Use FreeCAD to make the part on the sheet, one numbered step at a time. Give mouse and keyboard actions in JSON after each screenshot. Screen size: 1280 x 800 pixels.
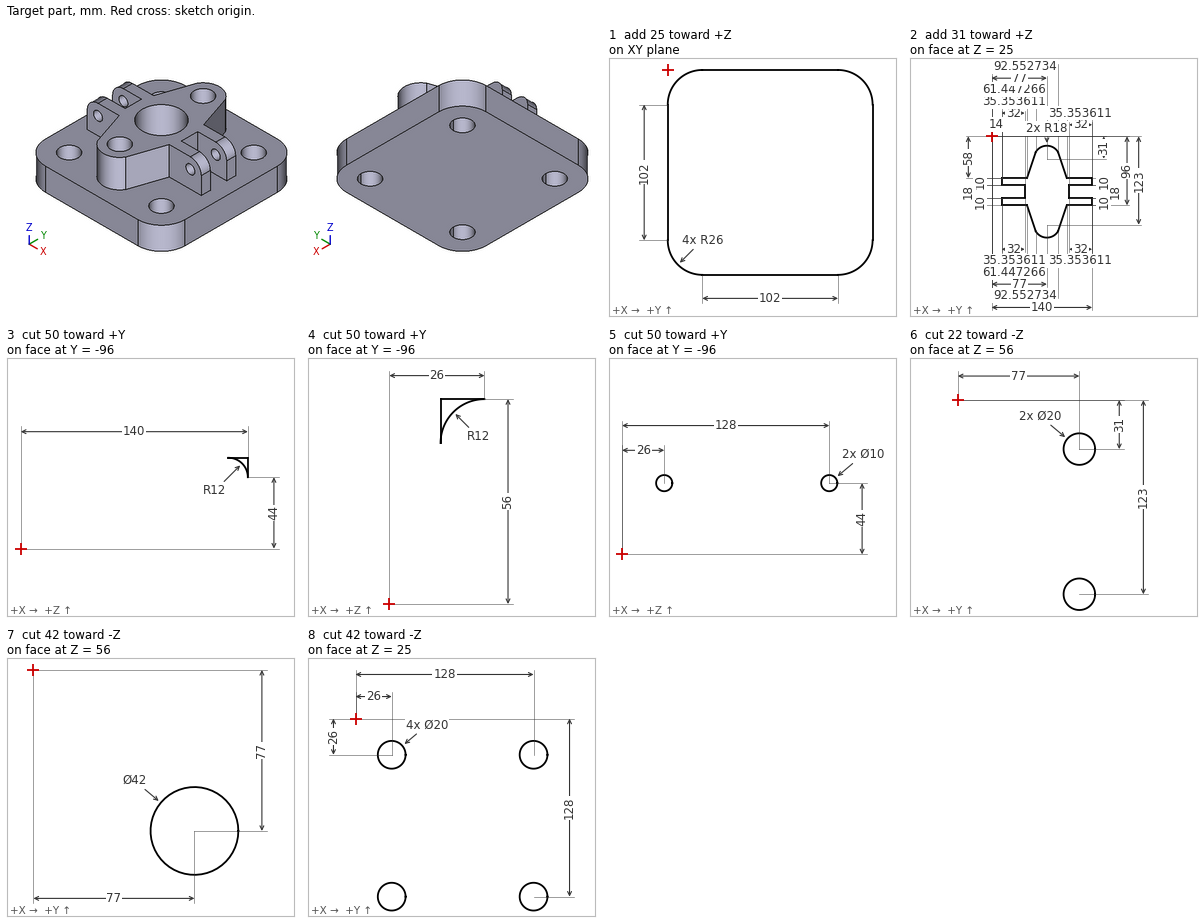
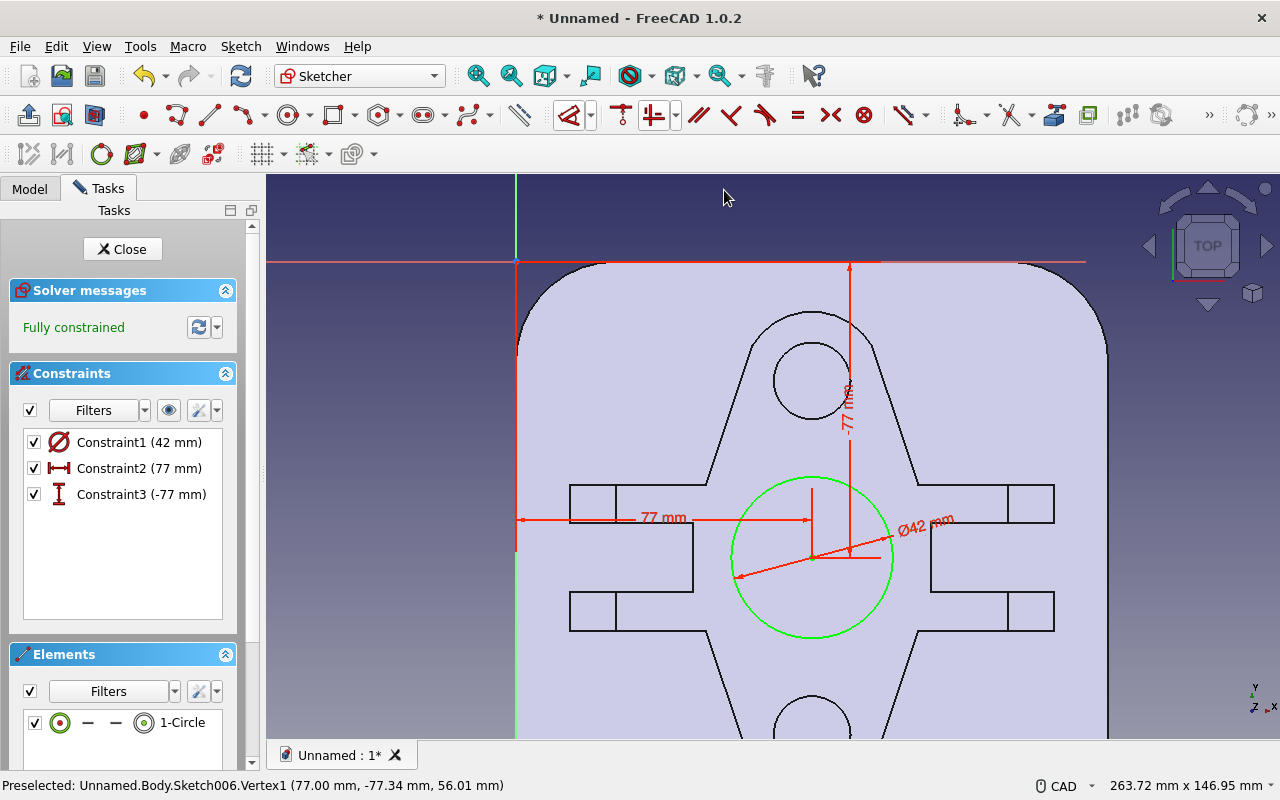
{"action": "left_click", "coordinate": [123, 249]}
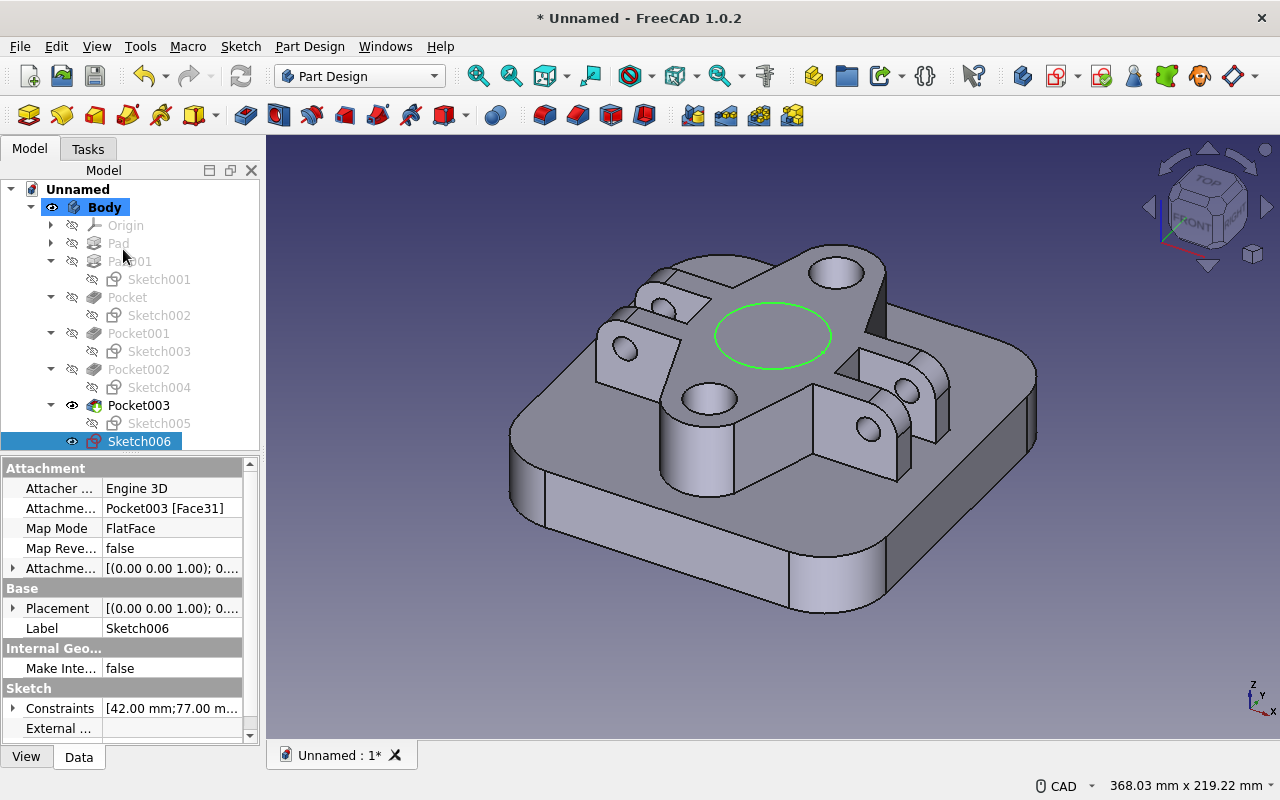
{"action": "left_click", "coordinate": [246, 116]}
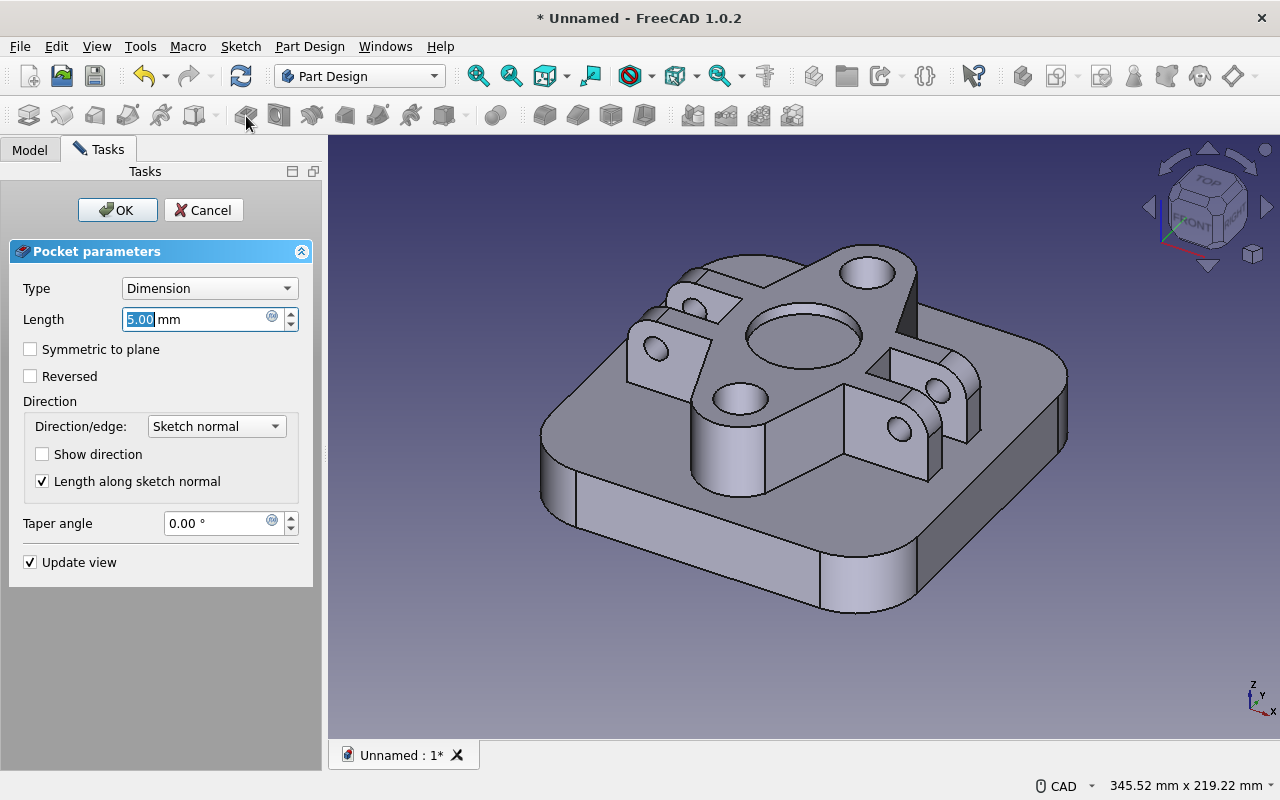
{"action": "type", "text": "42"}
{"action": "key", "text": "Tab"}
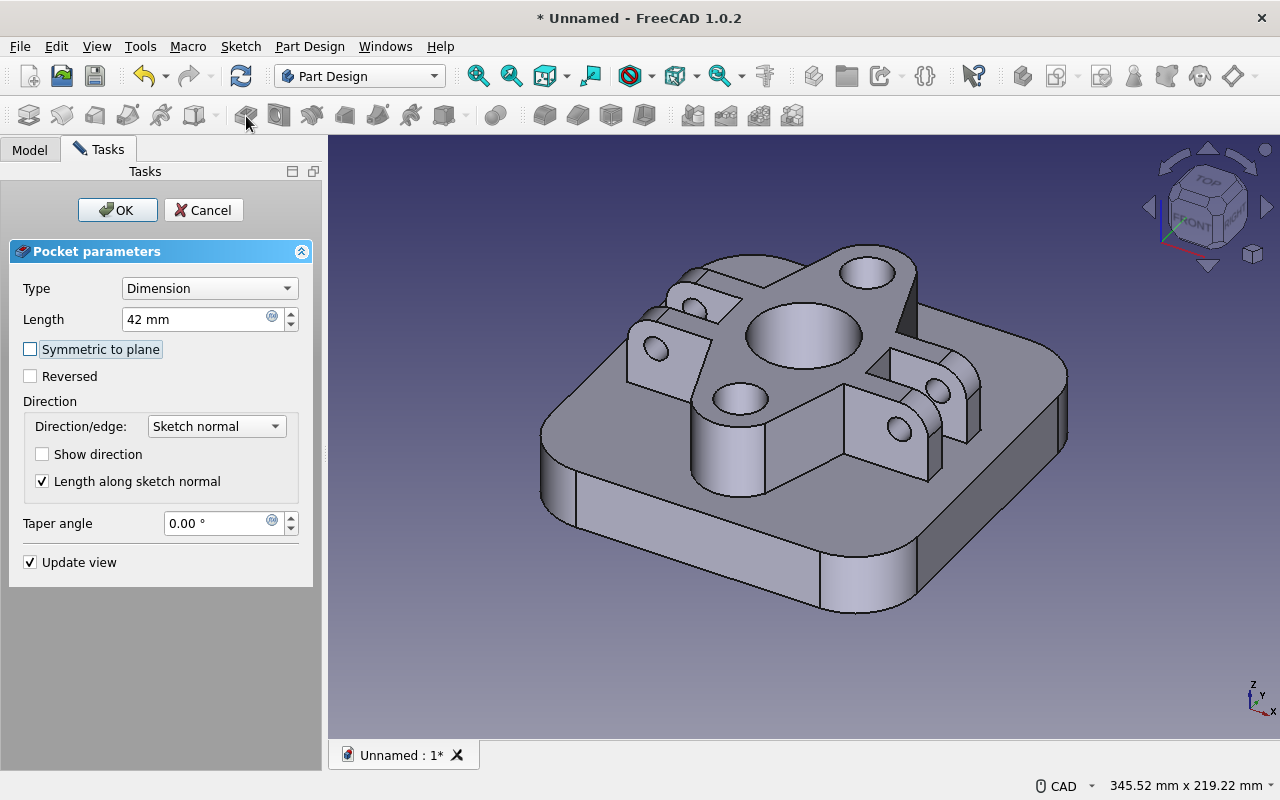
{"action": "left_click", "coordinate": [118, 210]}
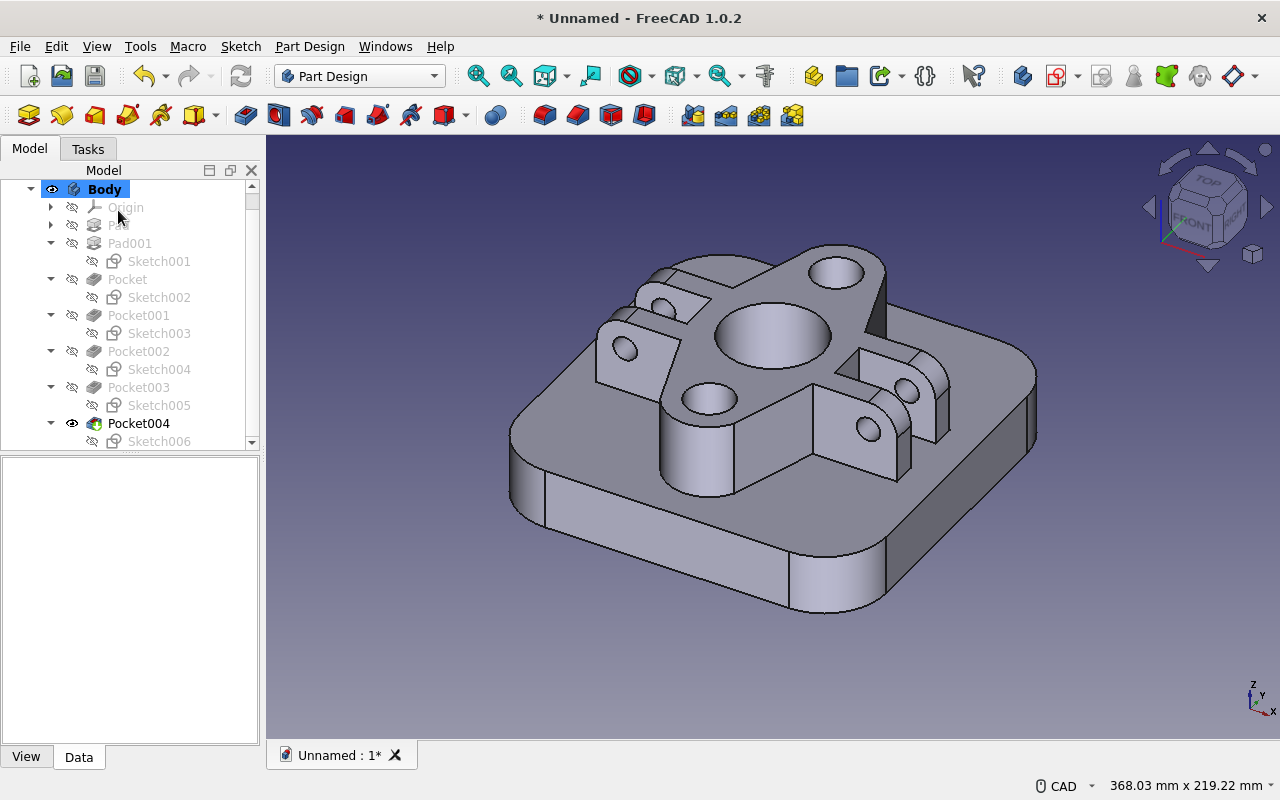
{"action": "left_click", "coordinate": [607, 430]}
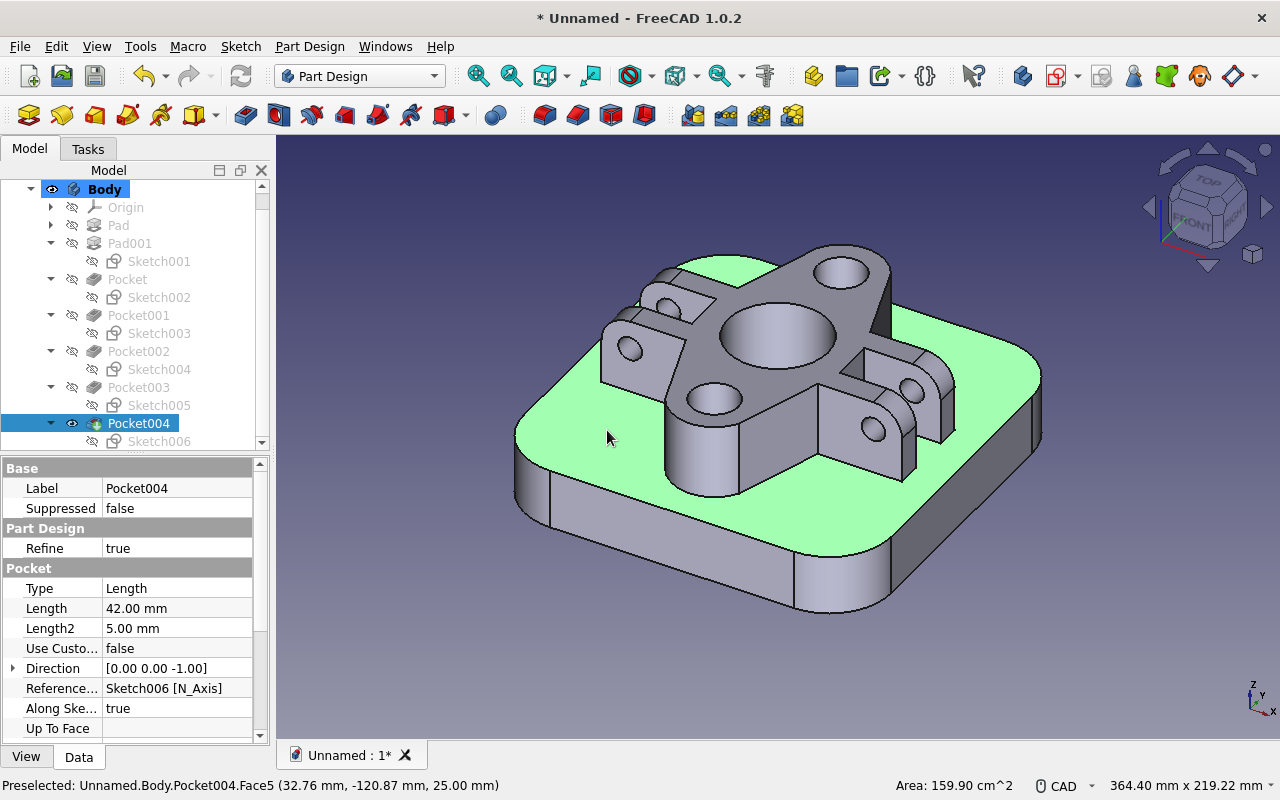
{"action": "left_click", "coordinate": [1056, 76]}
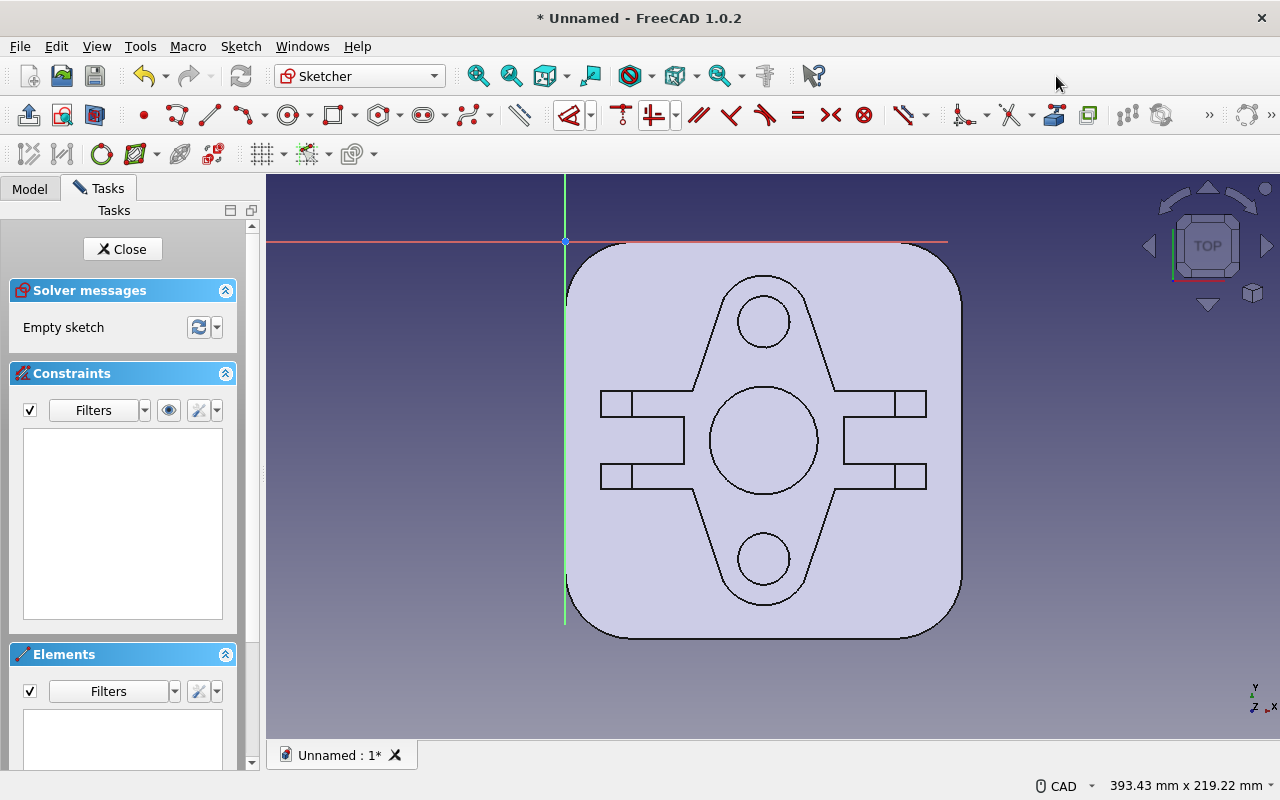
{"action": "left_click", "coordinate": [288, 116]}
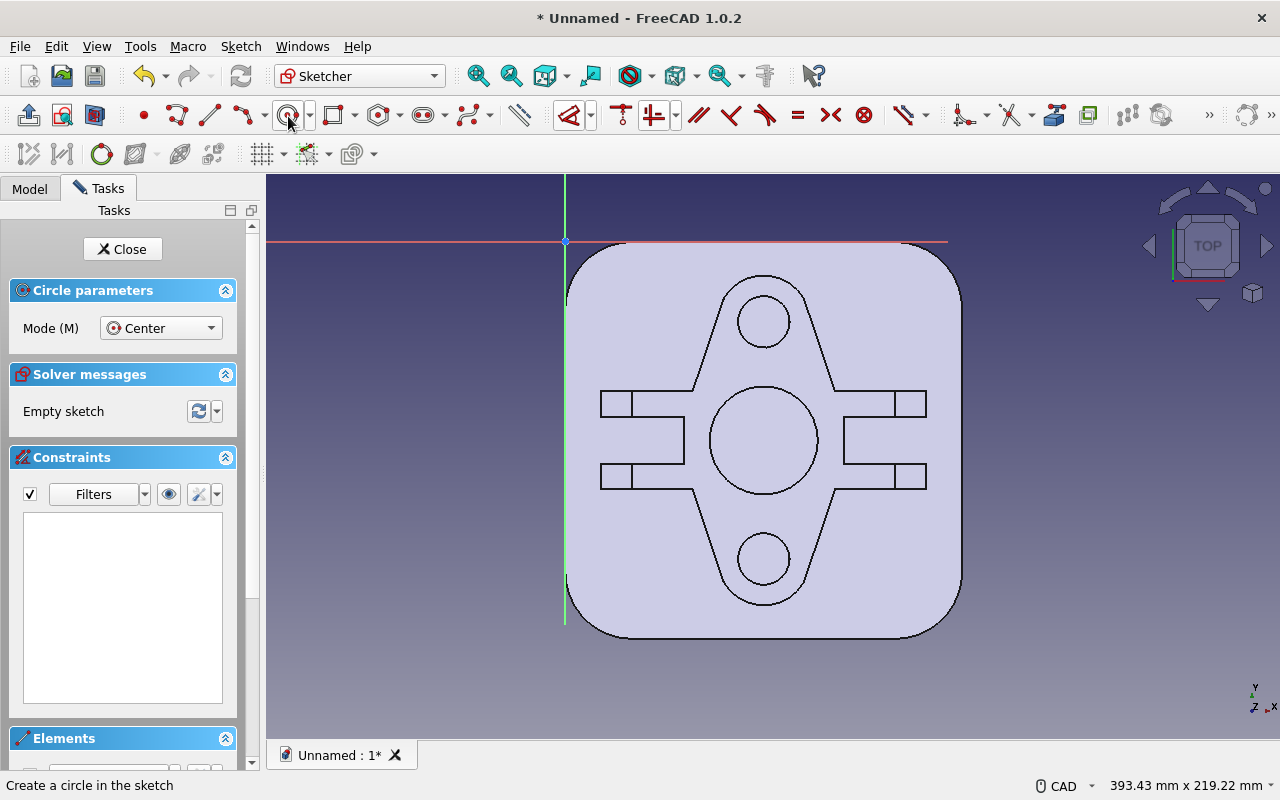
{"action": "left_click", "coordinate": [632, 309]}
{"action": "left_click", "coordinate": [651, 291]}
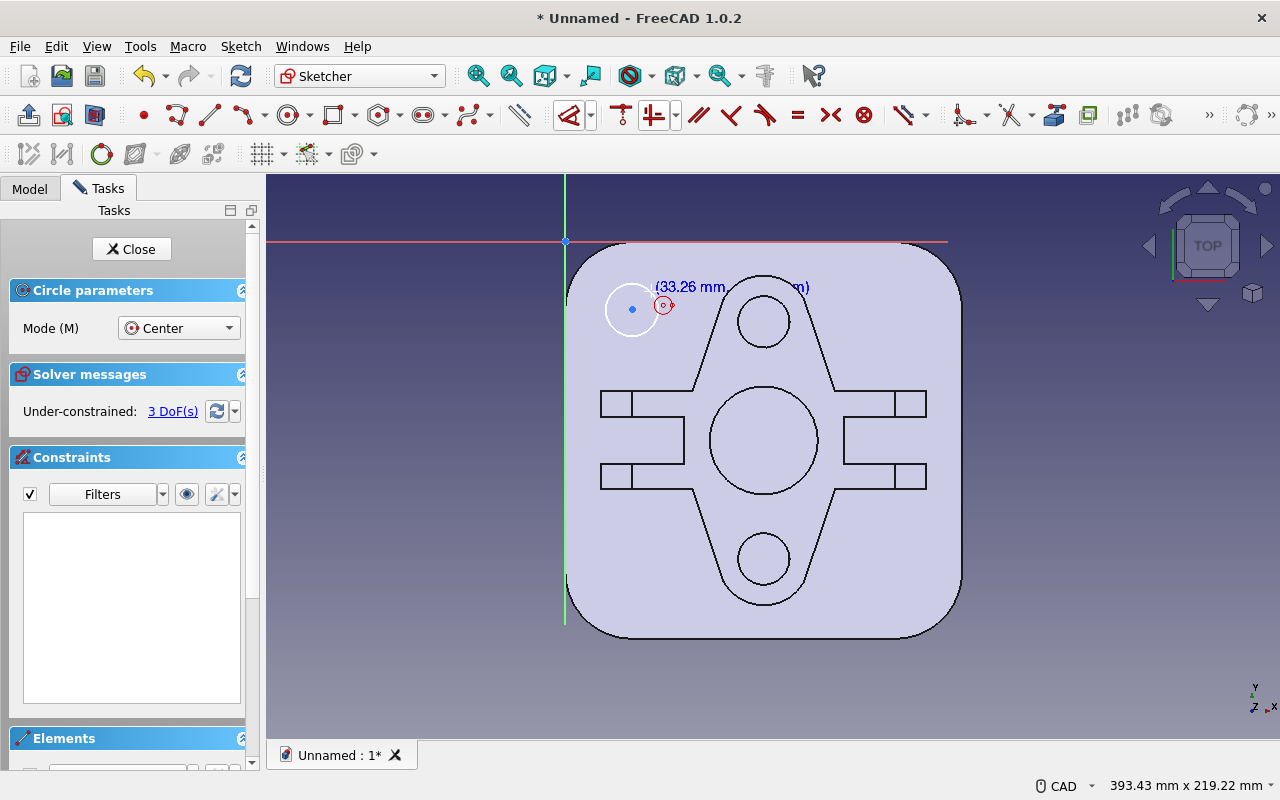
{"action": "left_click", "coordinate": [895, 309]}
{"action": "left_click", "coordinate": [913, 291]}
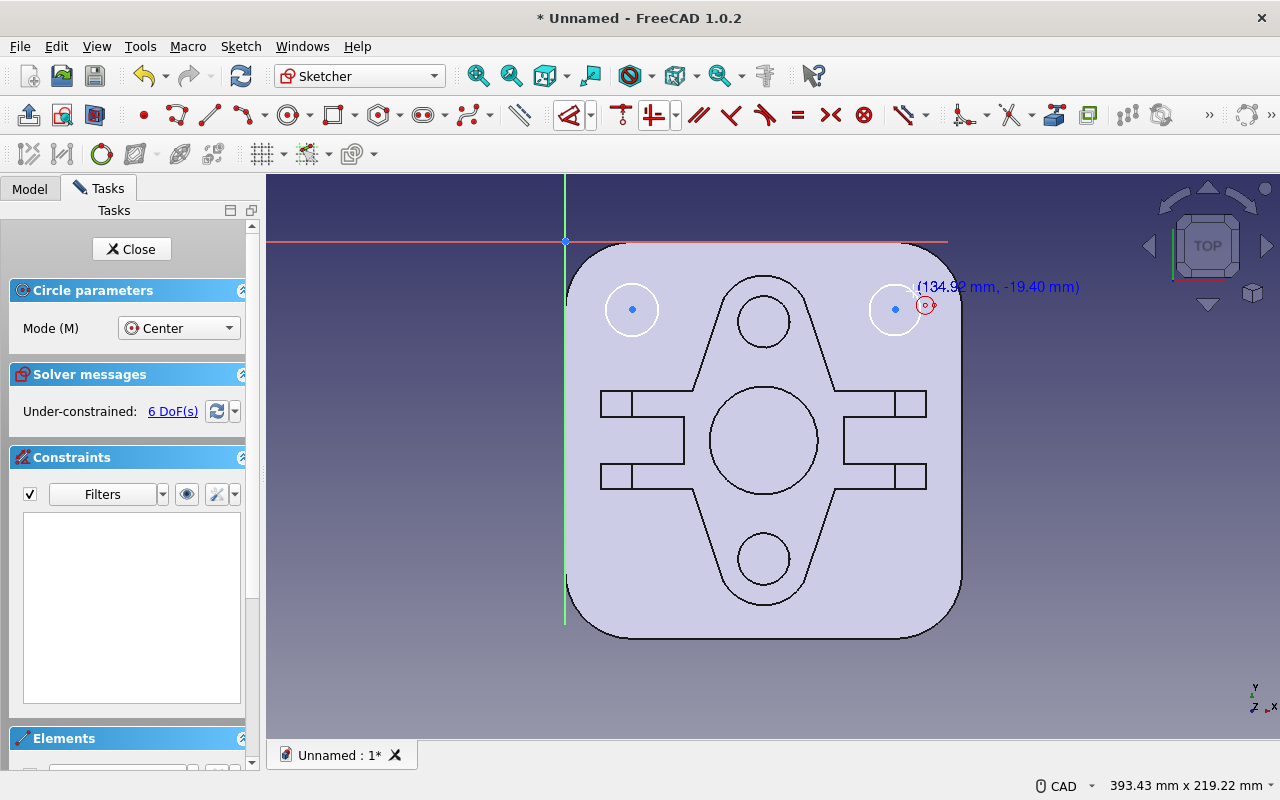
{"action": "left_click", "coordinate": [895, 572]}
{"action": "left_click", "coordinate": [913, 554]}